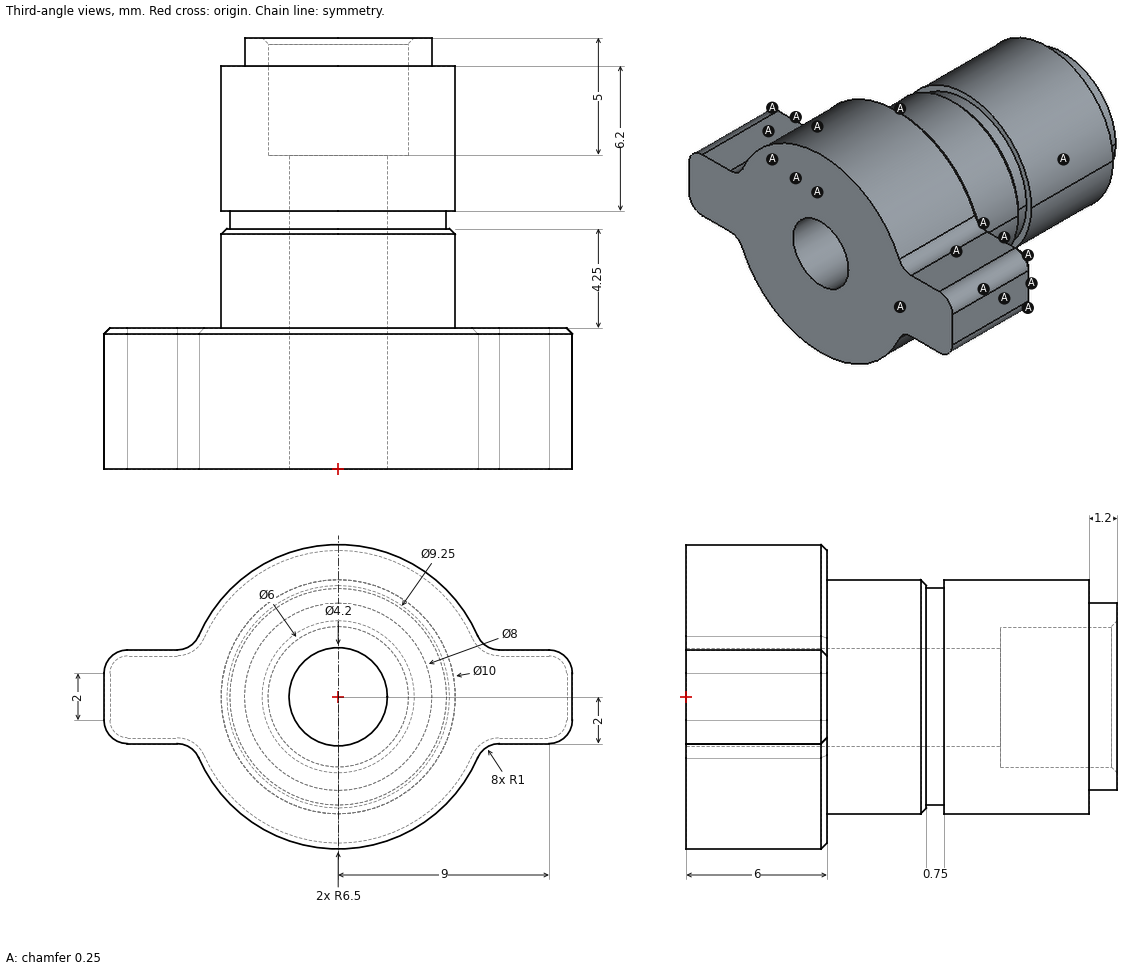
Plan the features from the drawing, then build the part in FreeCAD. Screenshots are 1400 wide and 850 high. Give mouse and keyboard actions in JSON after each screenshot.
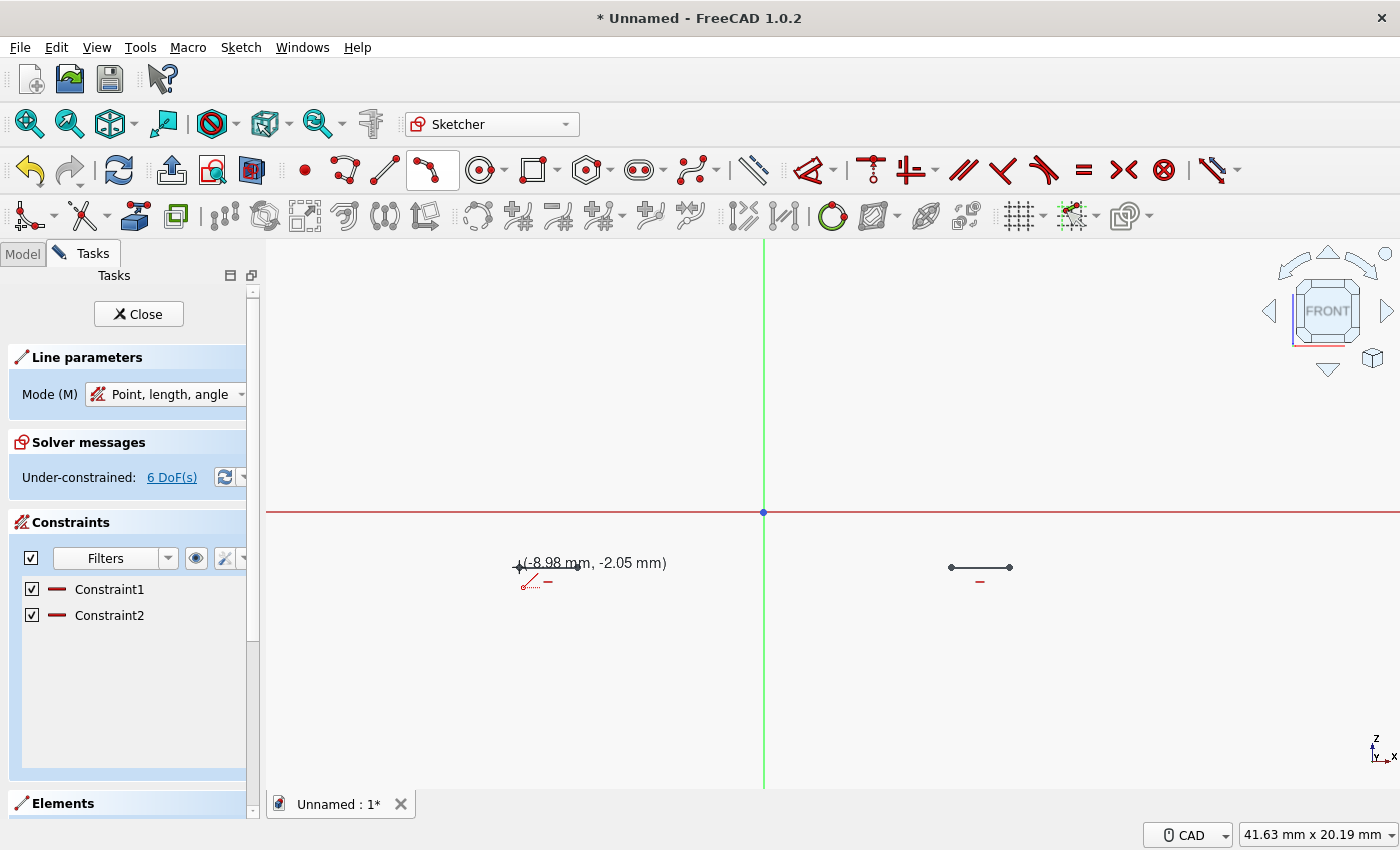
{"action": "left_click", "coordinate": [491, 539]}
{"action": "left_click", "coordinate": [491, 485]}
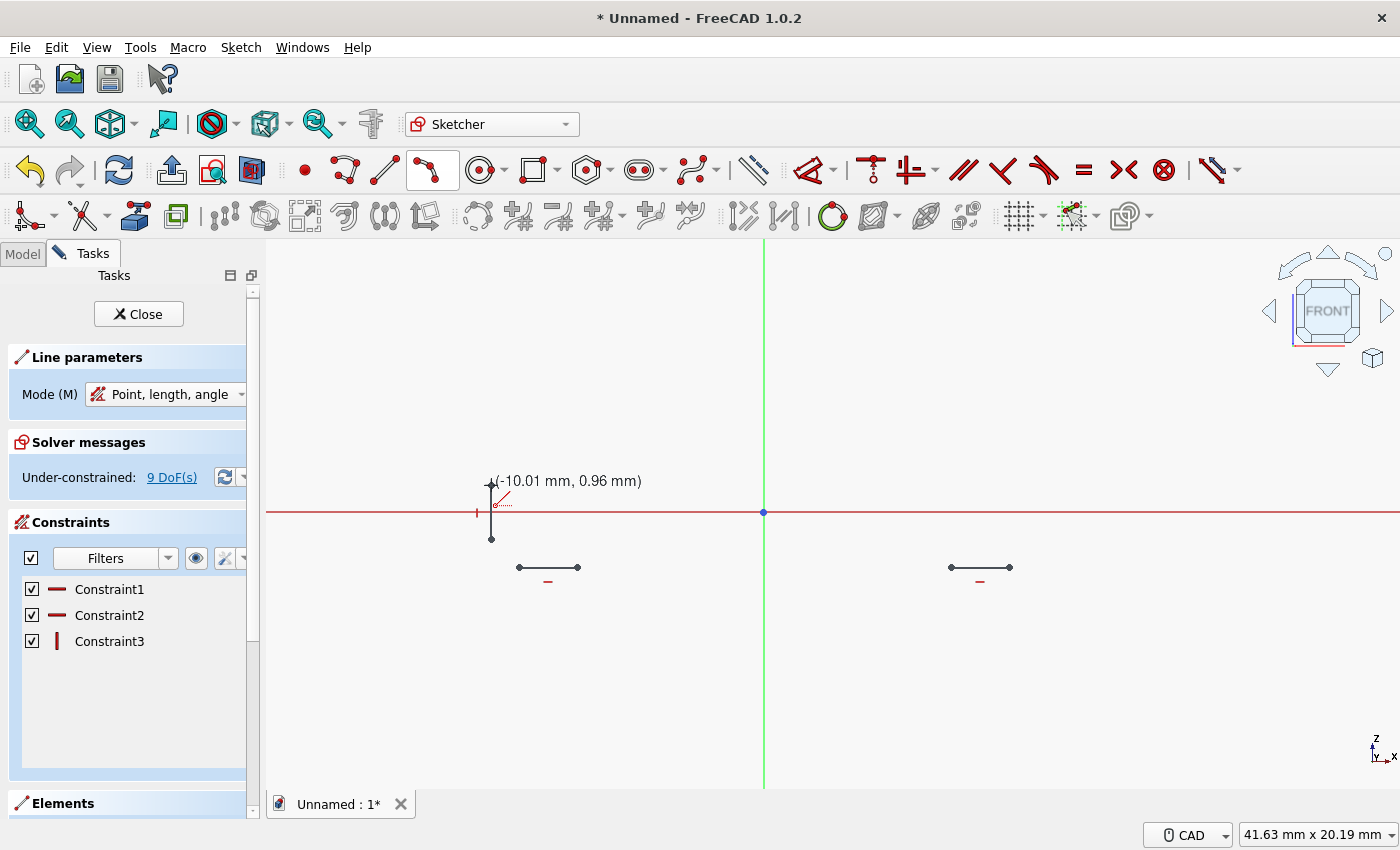
{"action": "left_click", "coordinate": [519, 458]}
{"action": "left_click", "coordinate": [577, 458]}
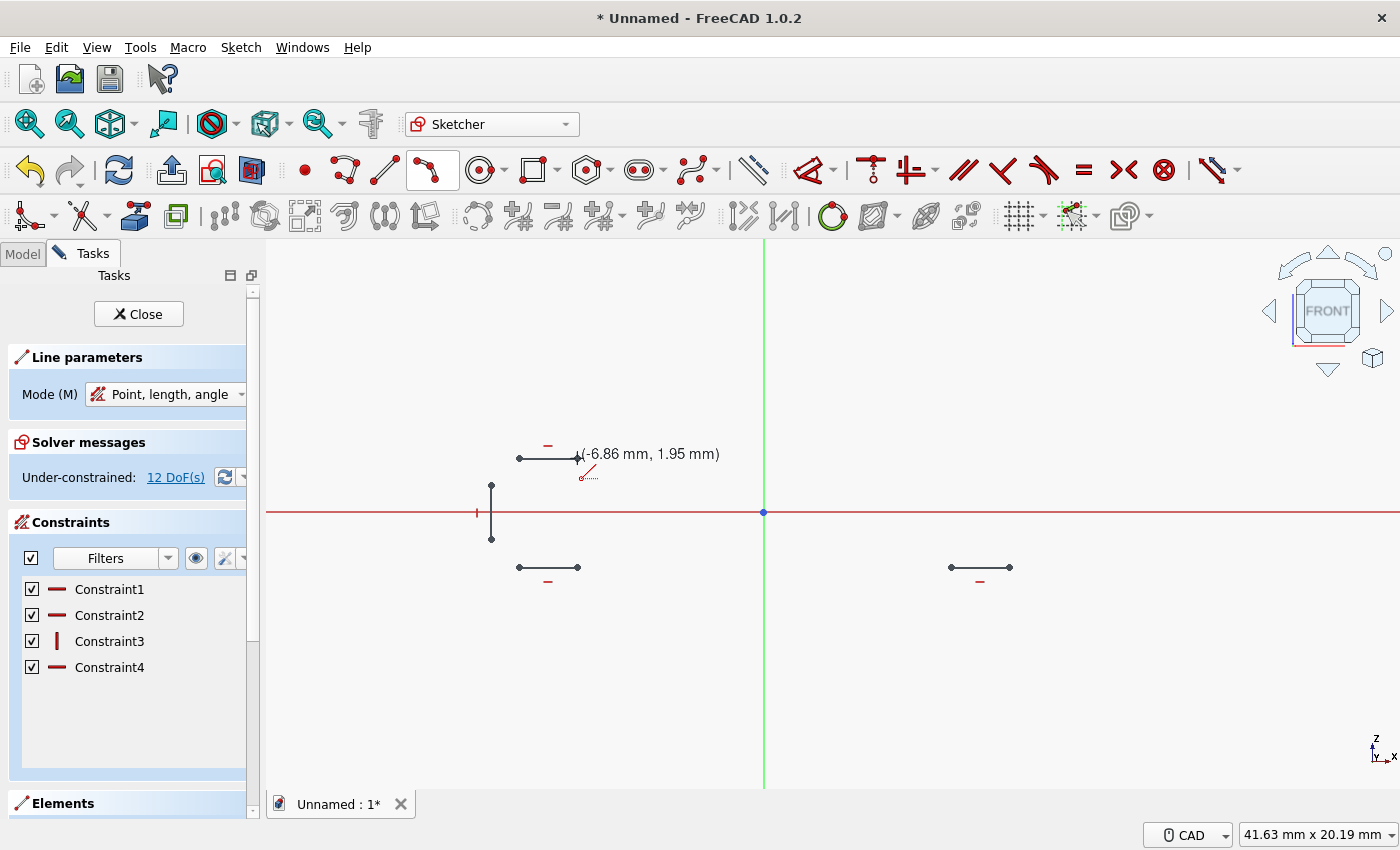
{"action": "left_click", "coordinate": [951, 458]}
{"action": "left_click", "coordinate": [1009, 458]}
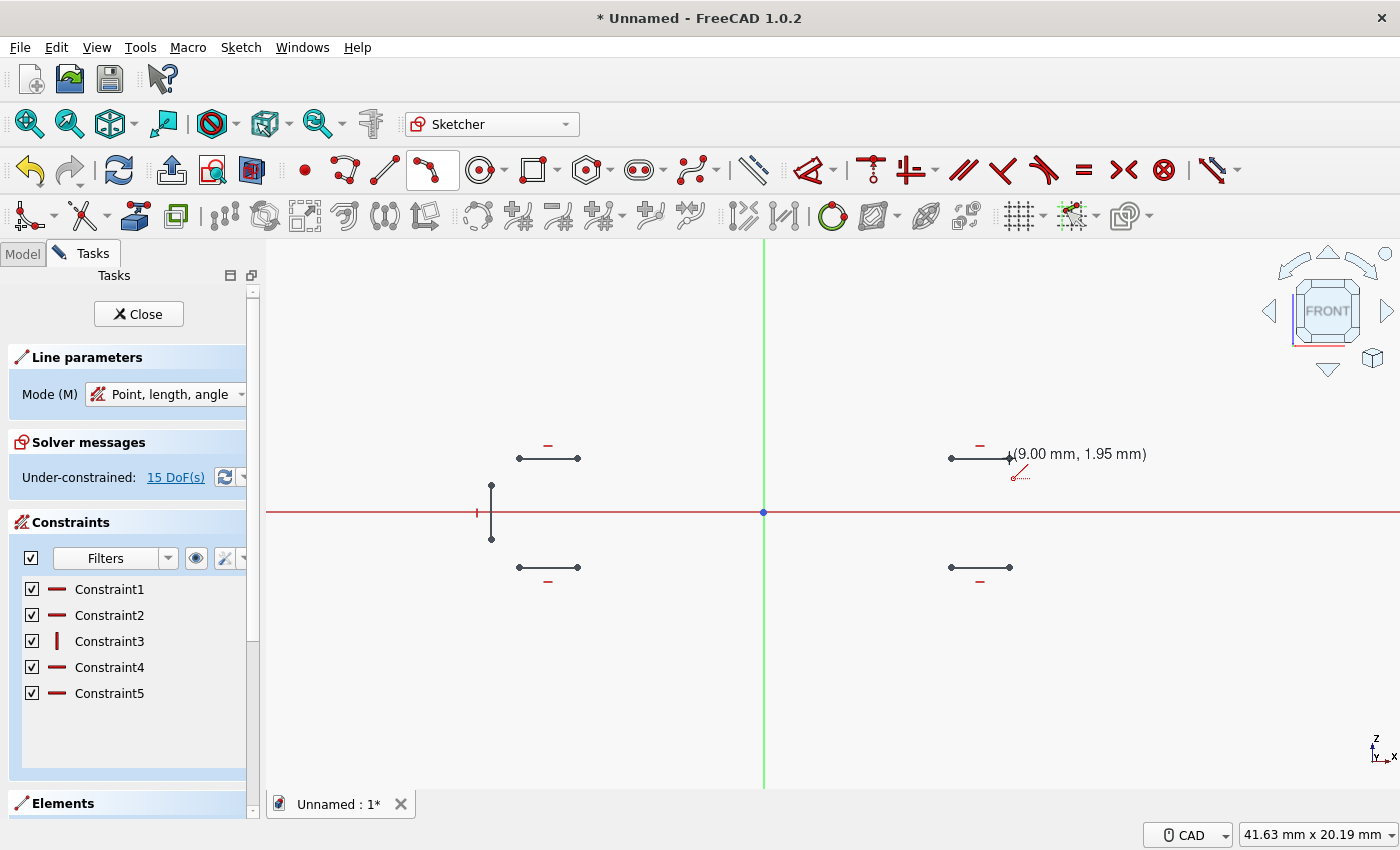
{"action": "left_click", "coordinate": [1036, 485]}
{"action": "left_click", "coordinate": [1036, 539]}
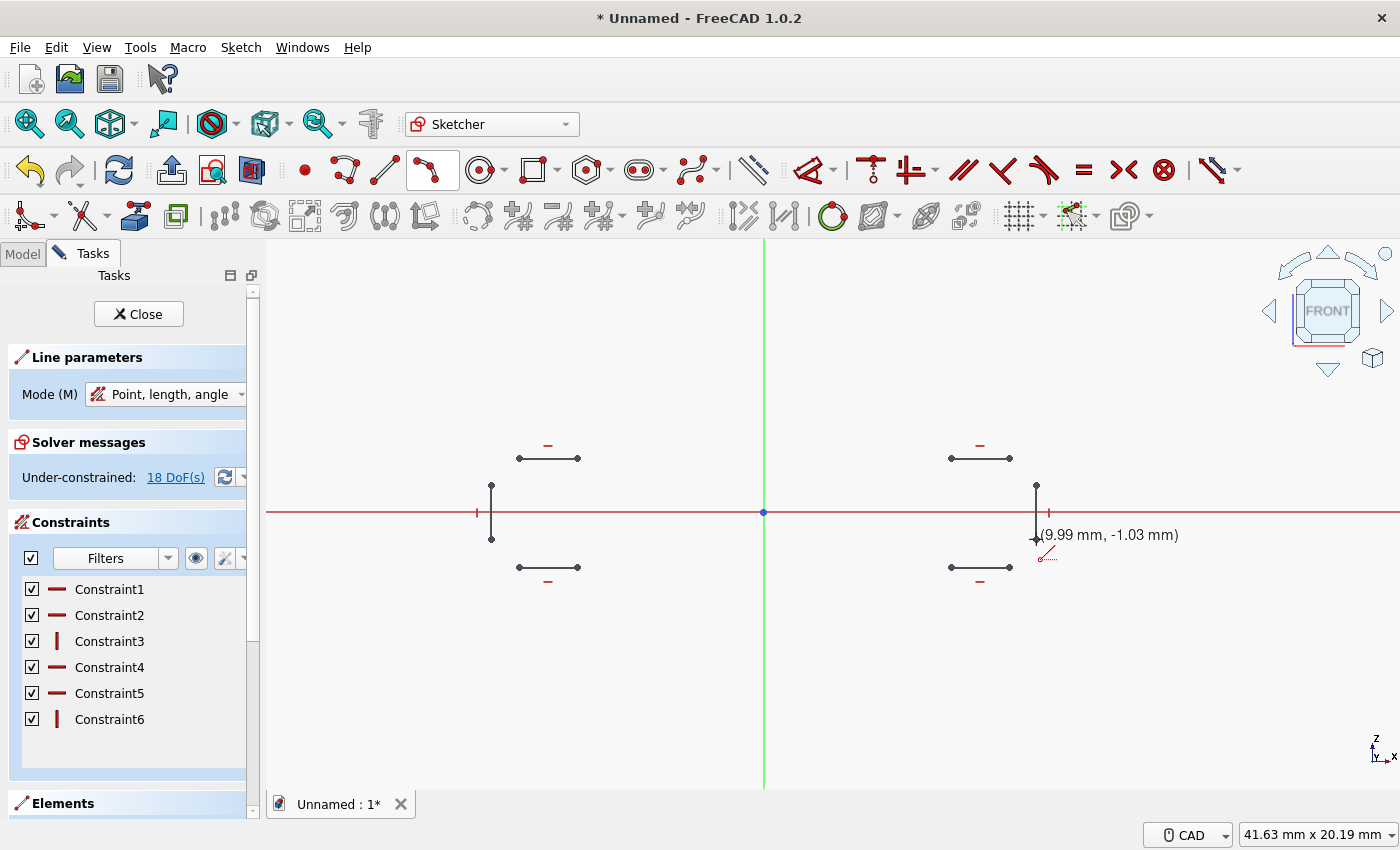
{"action": "left_click", "coordinate": [426, 170]}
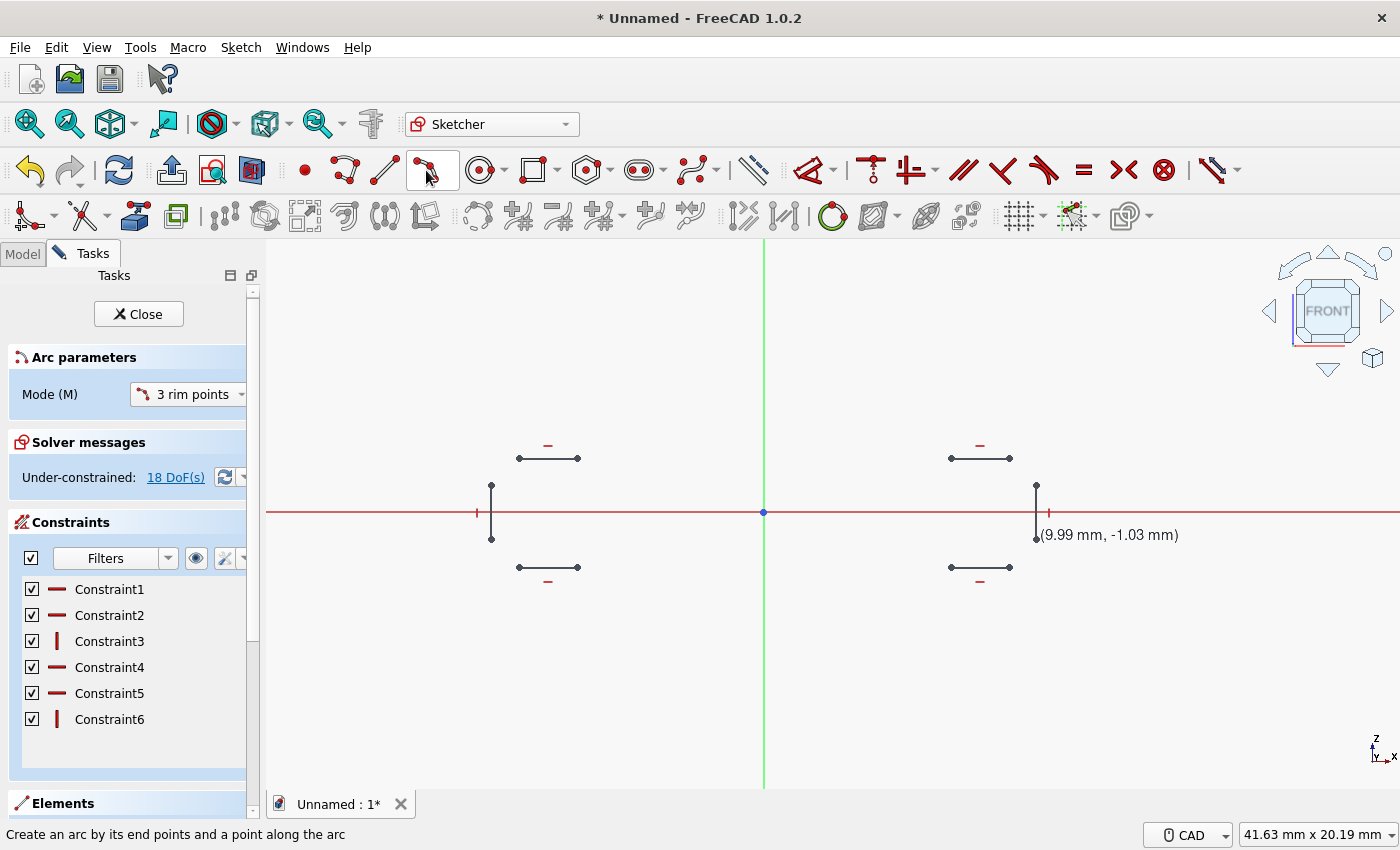
{"action": "left_click", "coordinate": [951, 568]}
{"action": "left_click", "coordinate": [926, 583]}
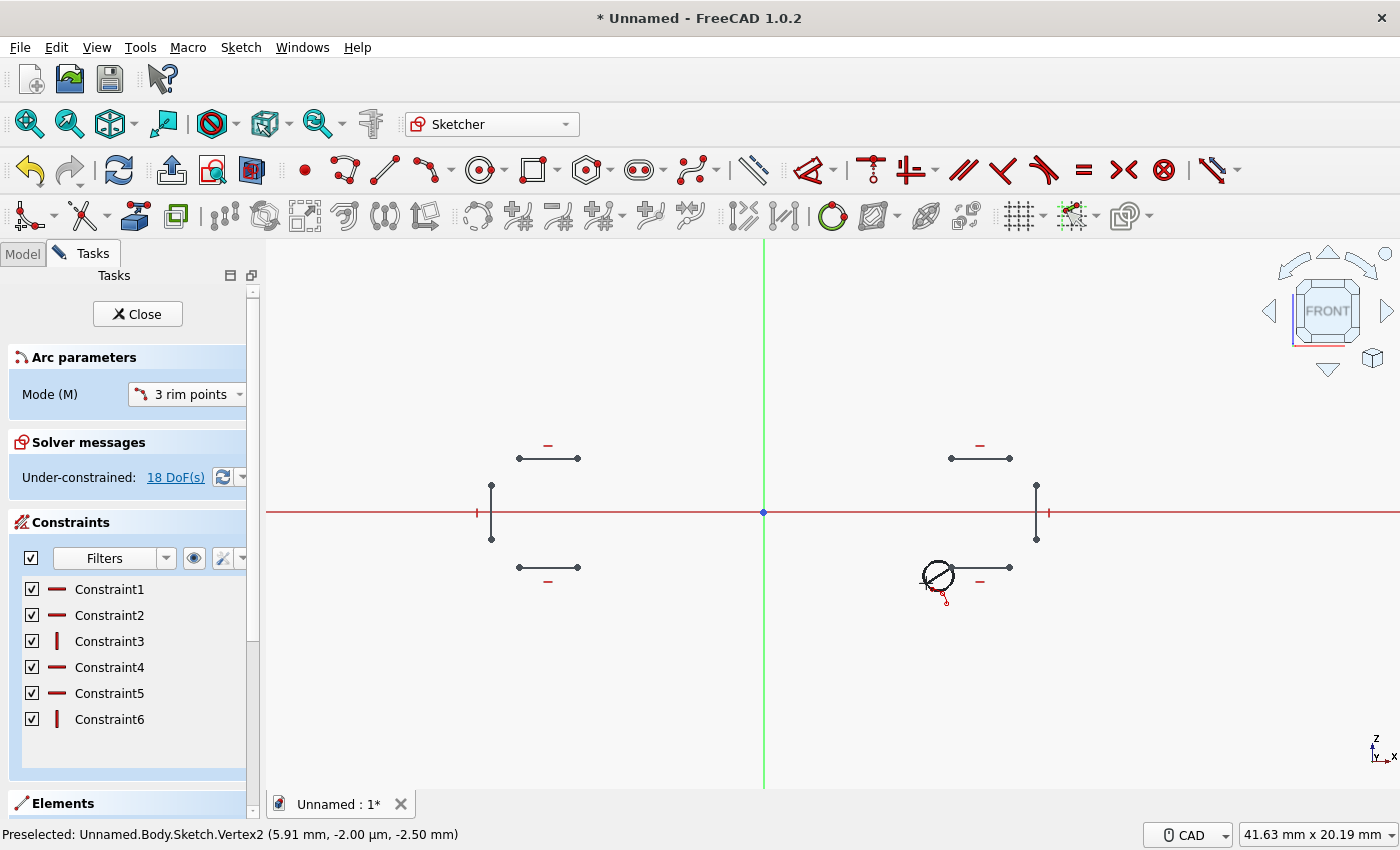
{"action": "scroll", "coordinate": [936, 571], "scroll_direction": "up", "scroll_amount": 7}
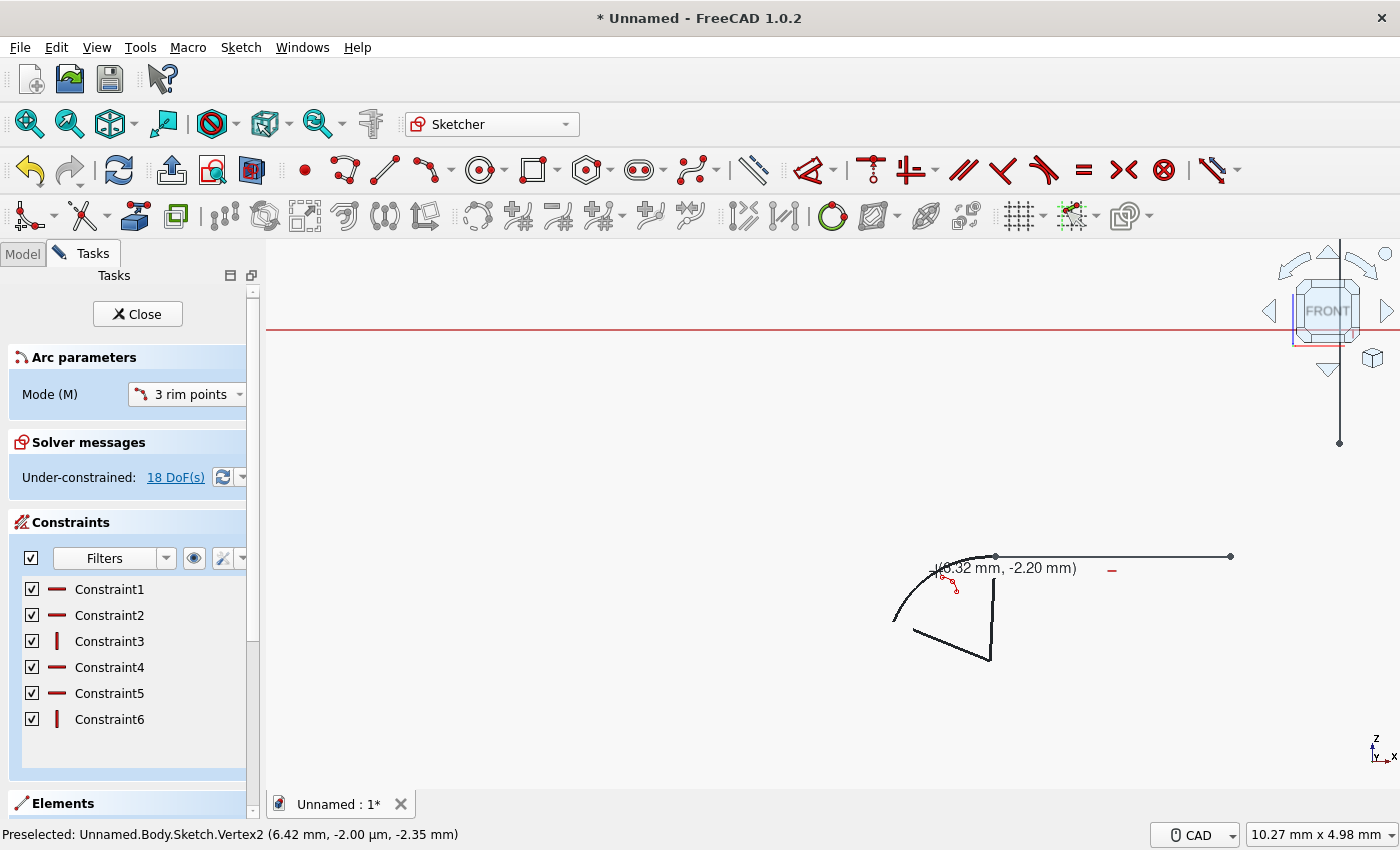
{"action": "left_click", "coordinate": [935, 569]}